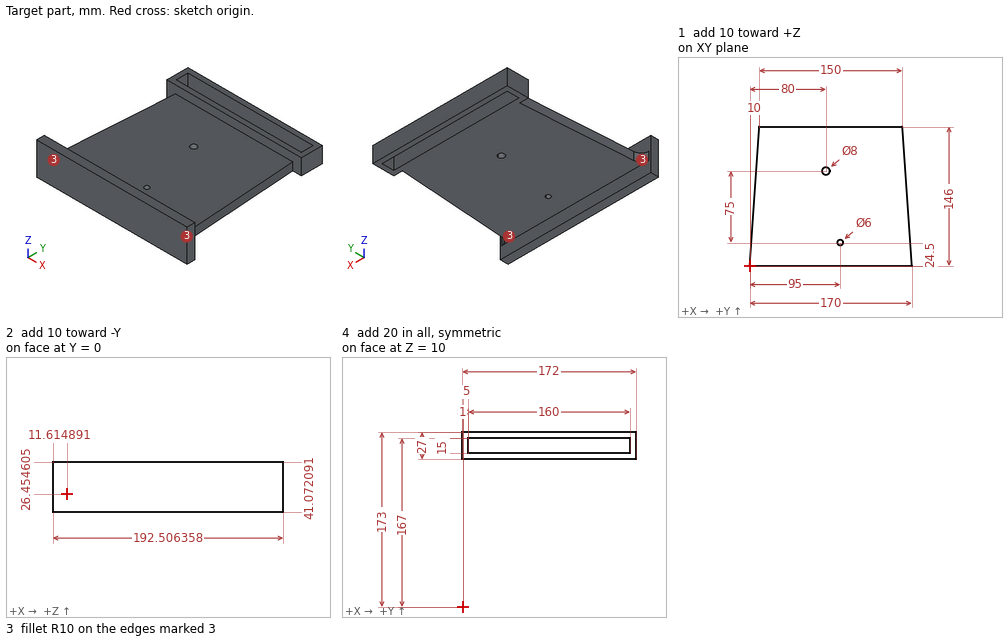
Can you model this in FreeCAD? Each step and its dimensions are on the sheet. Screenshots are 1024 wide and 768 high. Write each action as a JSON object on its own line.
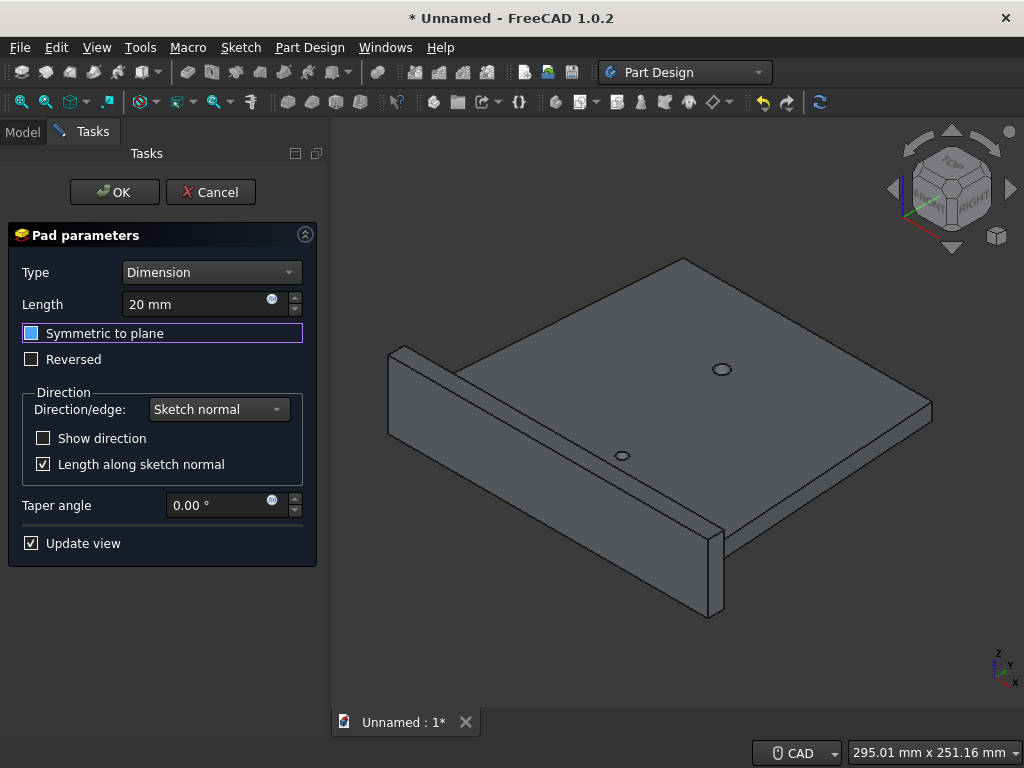
{"action": "left_click", "coordinate": [30, 333]}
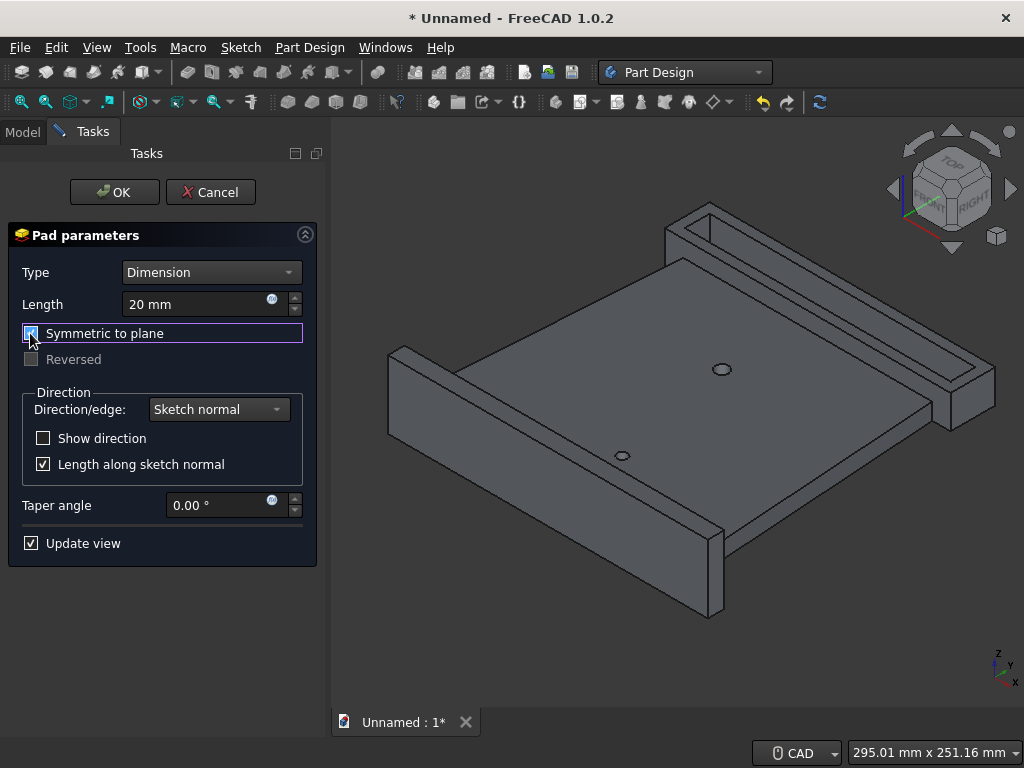
{"action": "left_click", "coordinate": [115, 192]}